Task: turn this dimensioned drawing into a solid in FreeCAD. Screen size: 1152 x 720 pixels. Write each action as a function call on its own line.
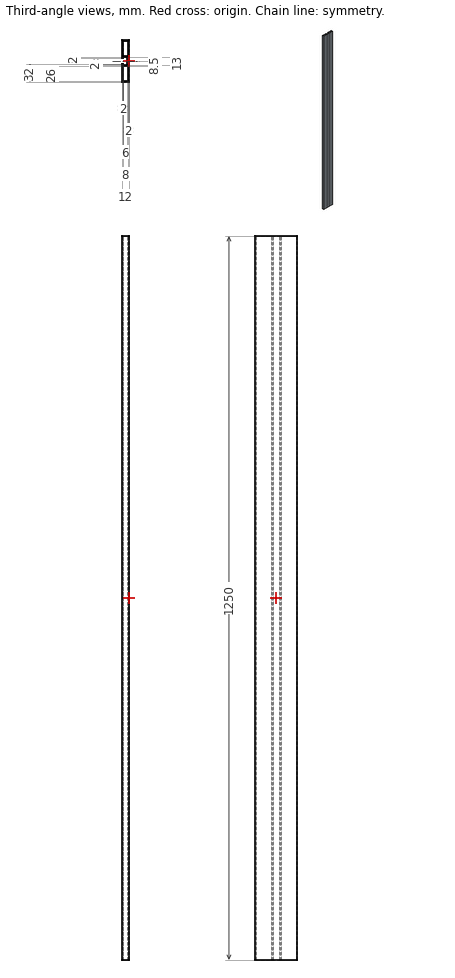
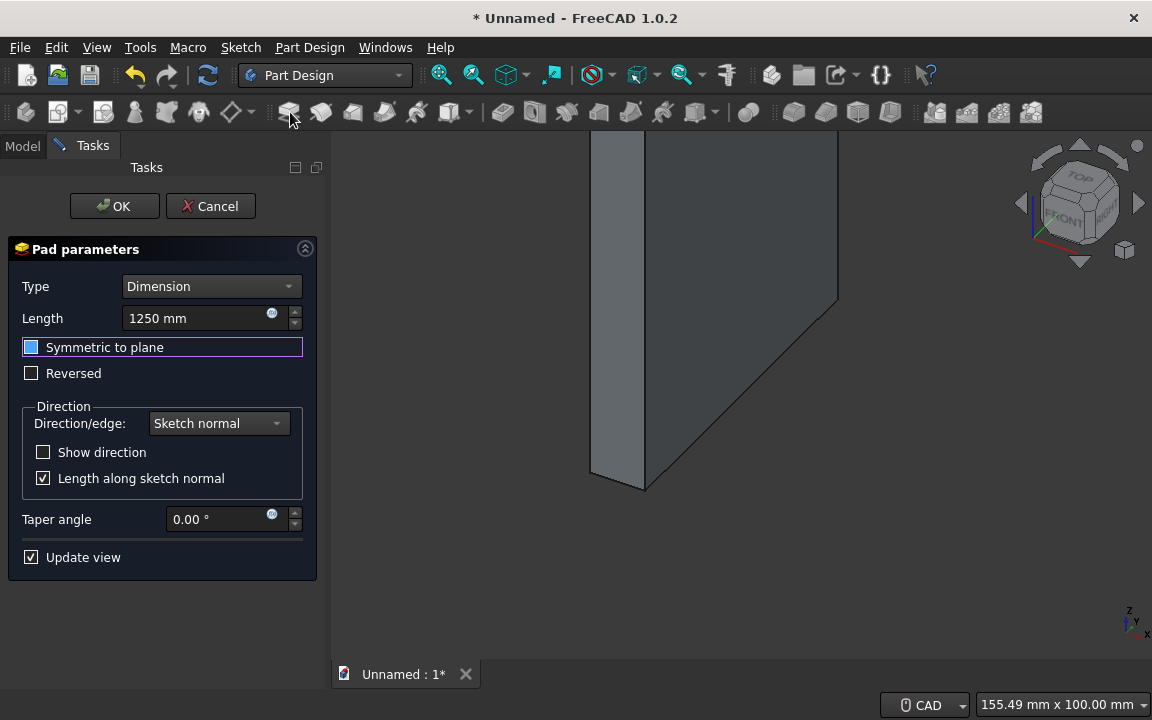
click(30, 347)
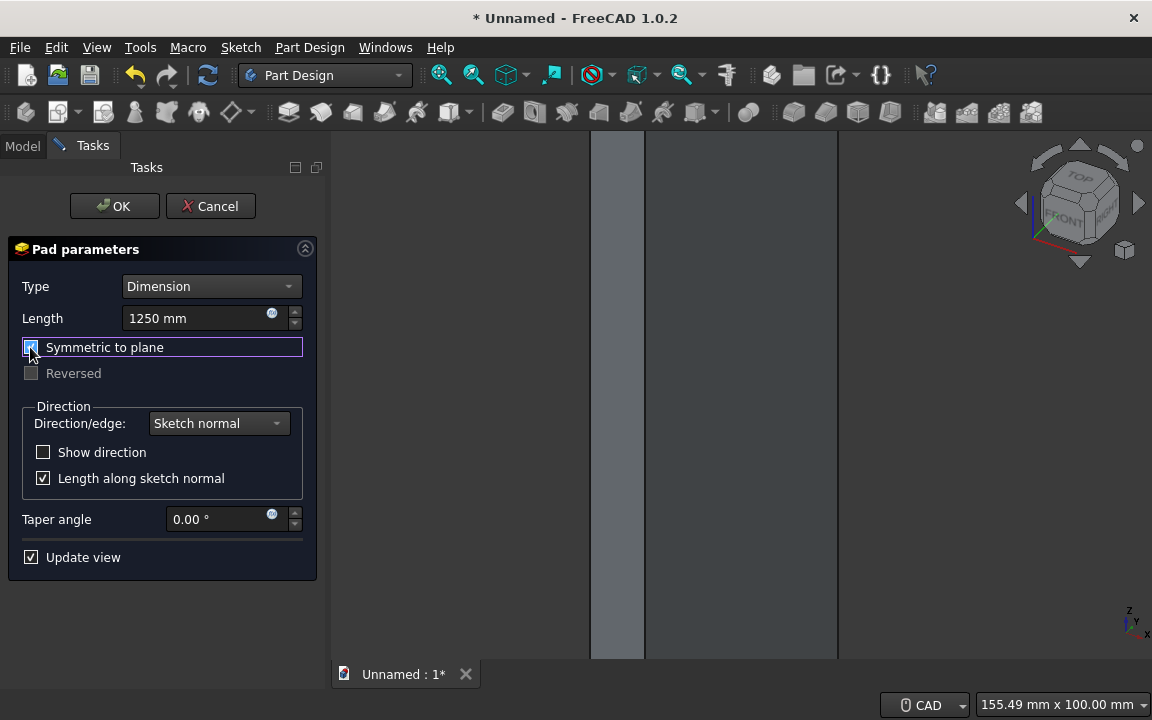
click(115, 206)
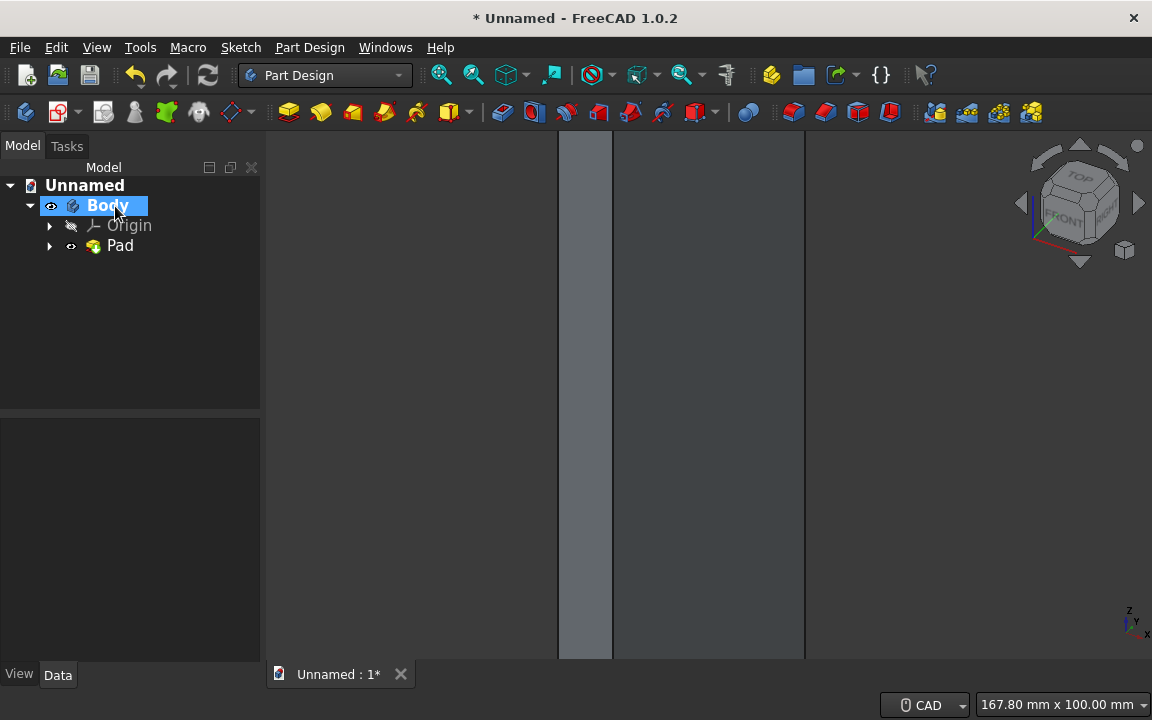
key(0)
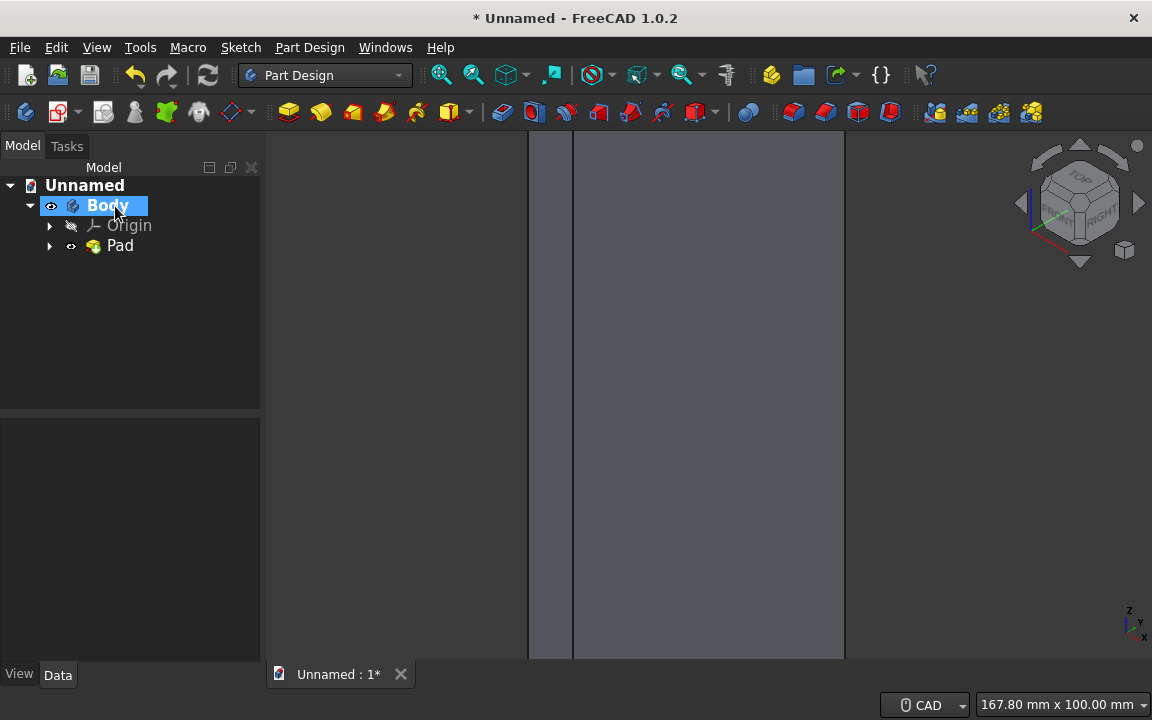
click(442, 76)